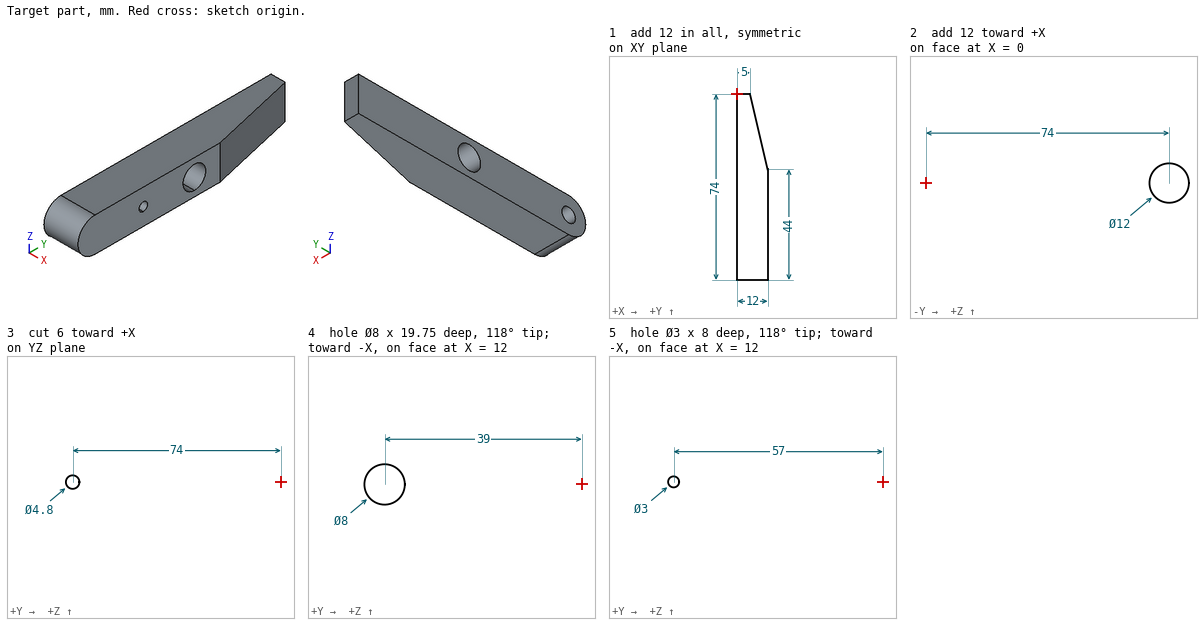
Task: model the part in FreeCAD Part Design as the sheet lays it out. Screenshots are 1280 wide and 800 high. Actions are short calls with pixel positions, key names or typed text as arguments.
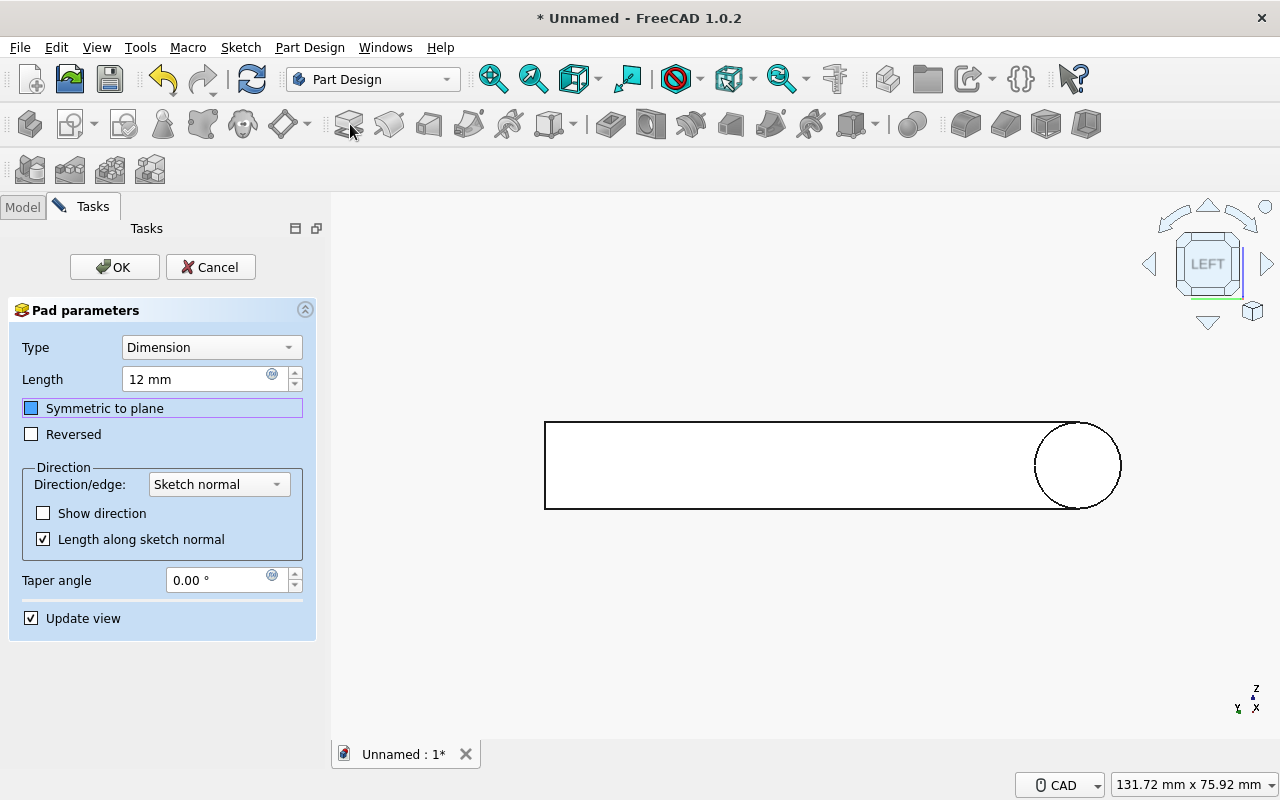
click(30, 434)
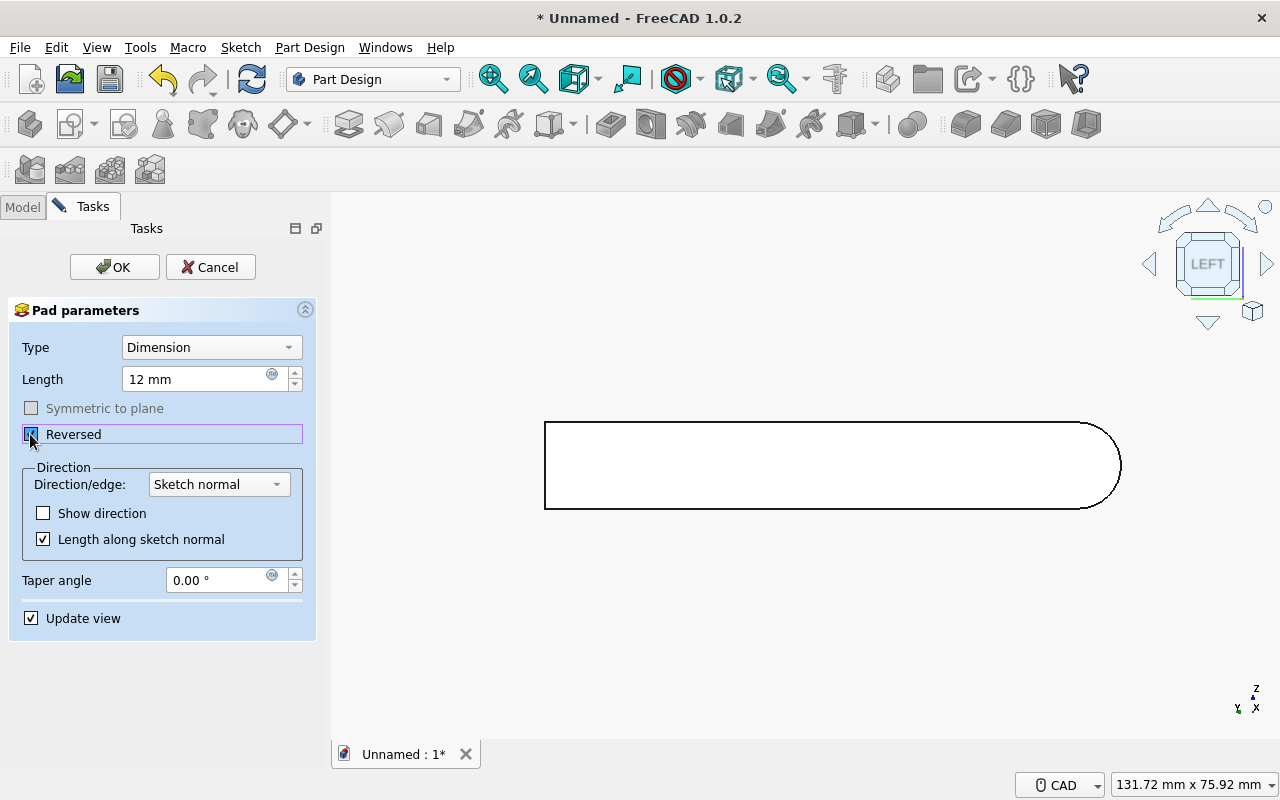
click(115, 267)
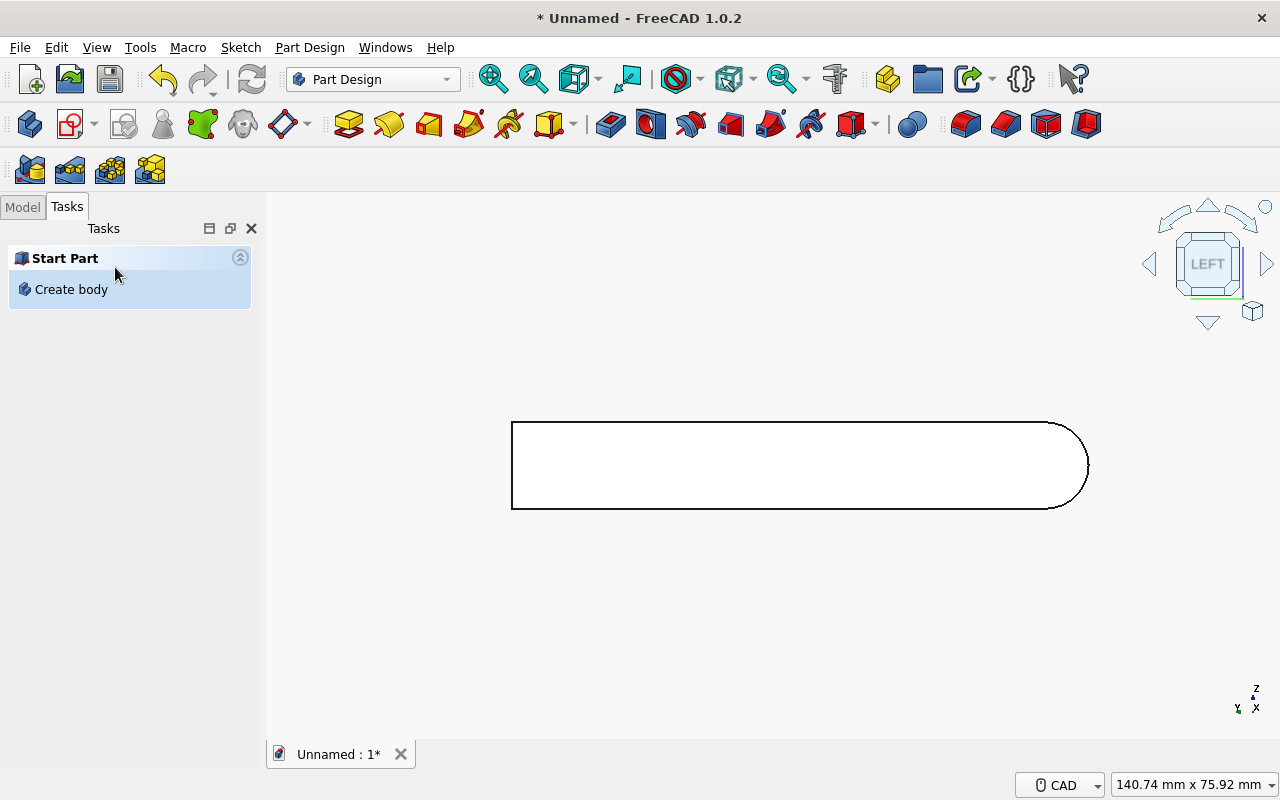
click(70, 124)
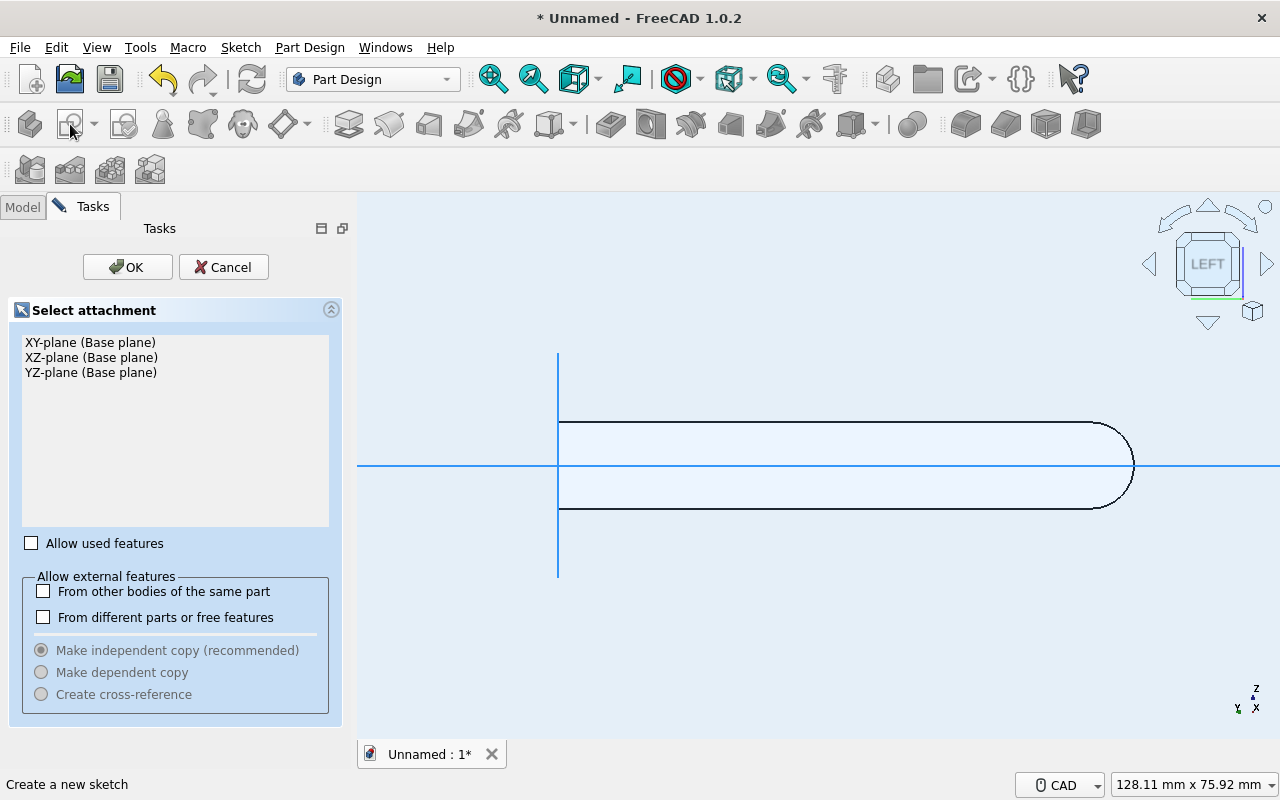
click(82, 372)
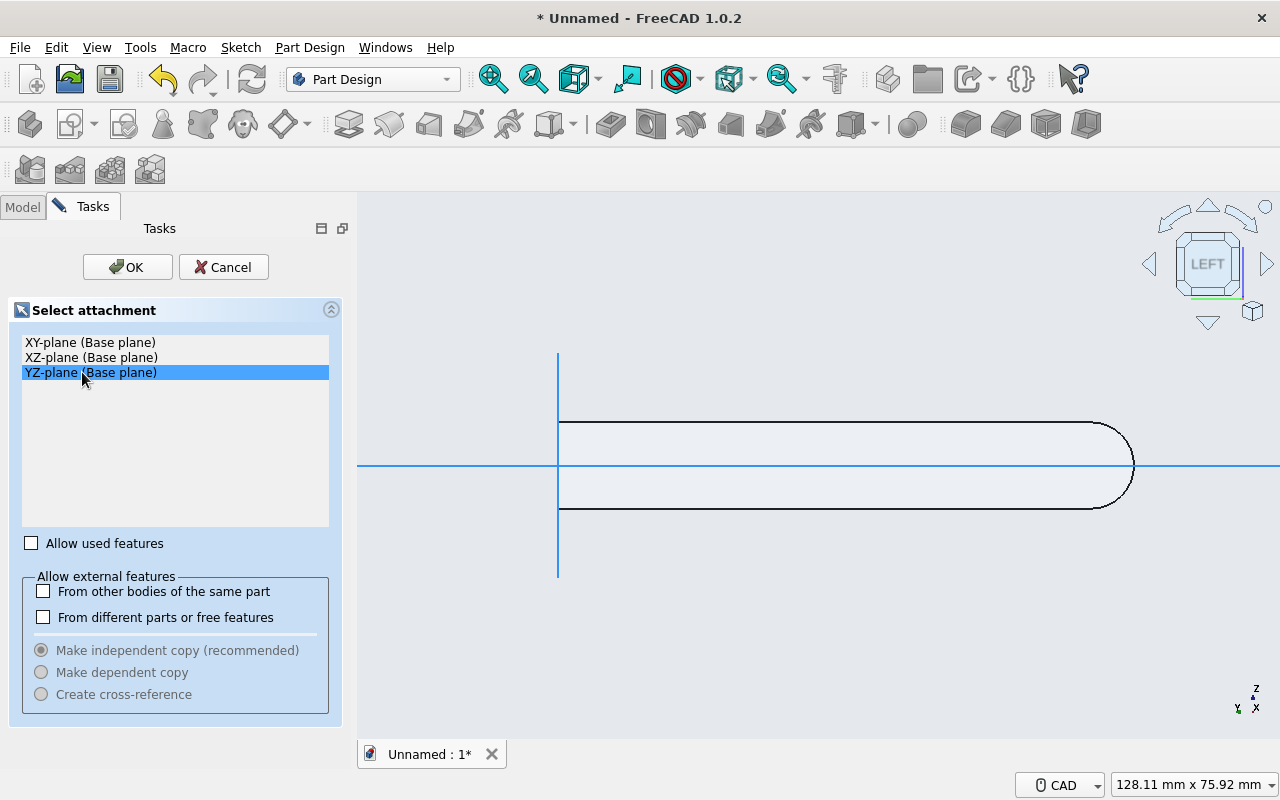
click(128, 267)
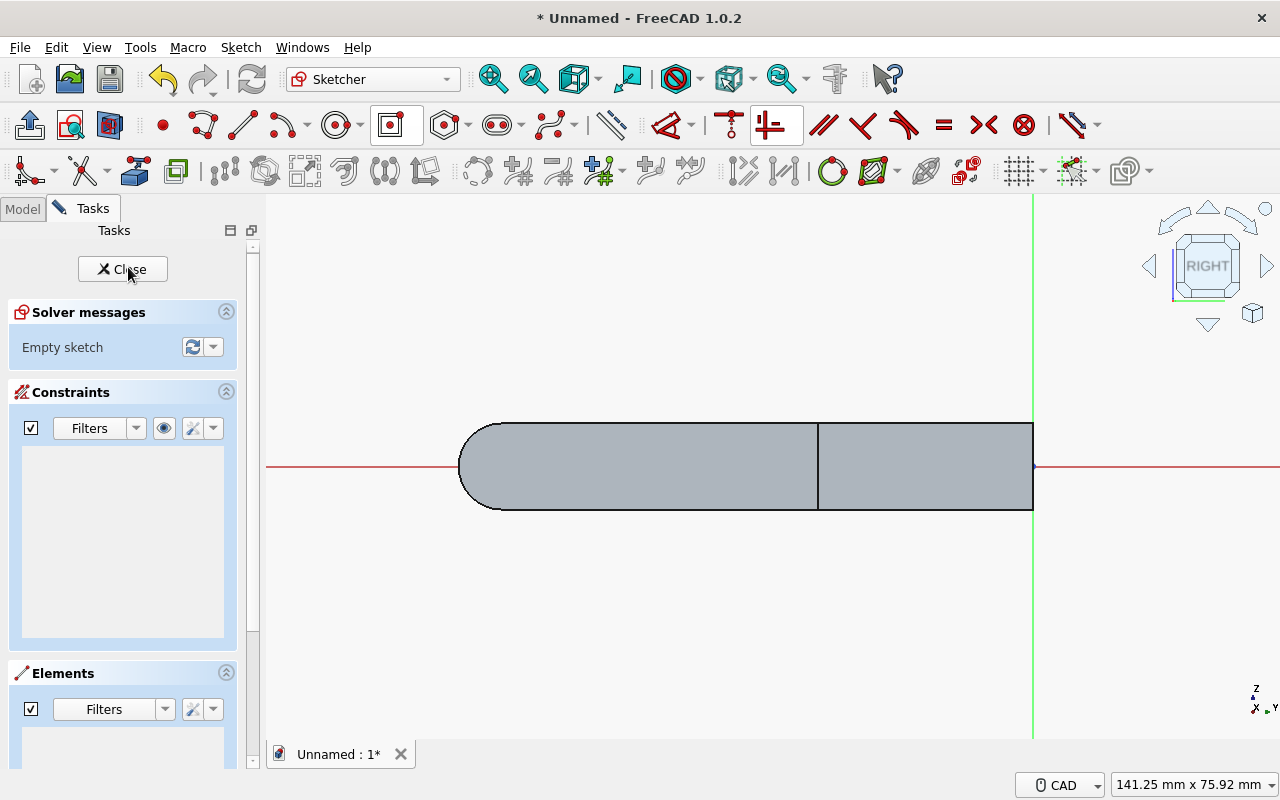
click(110, 126)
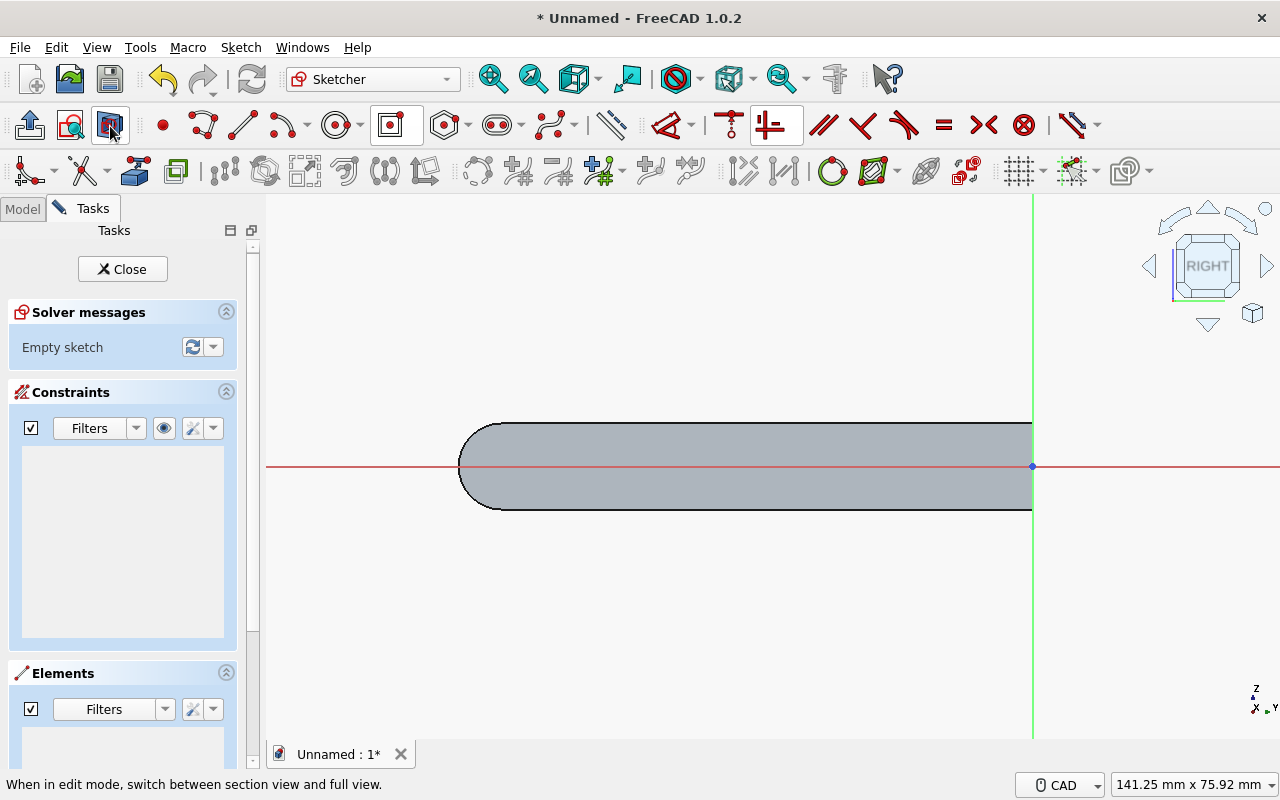
scroll(481, 467, up, 12)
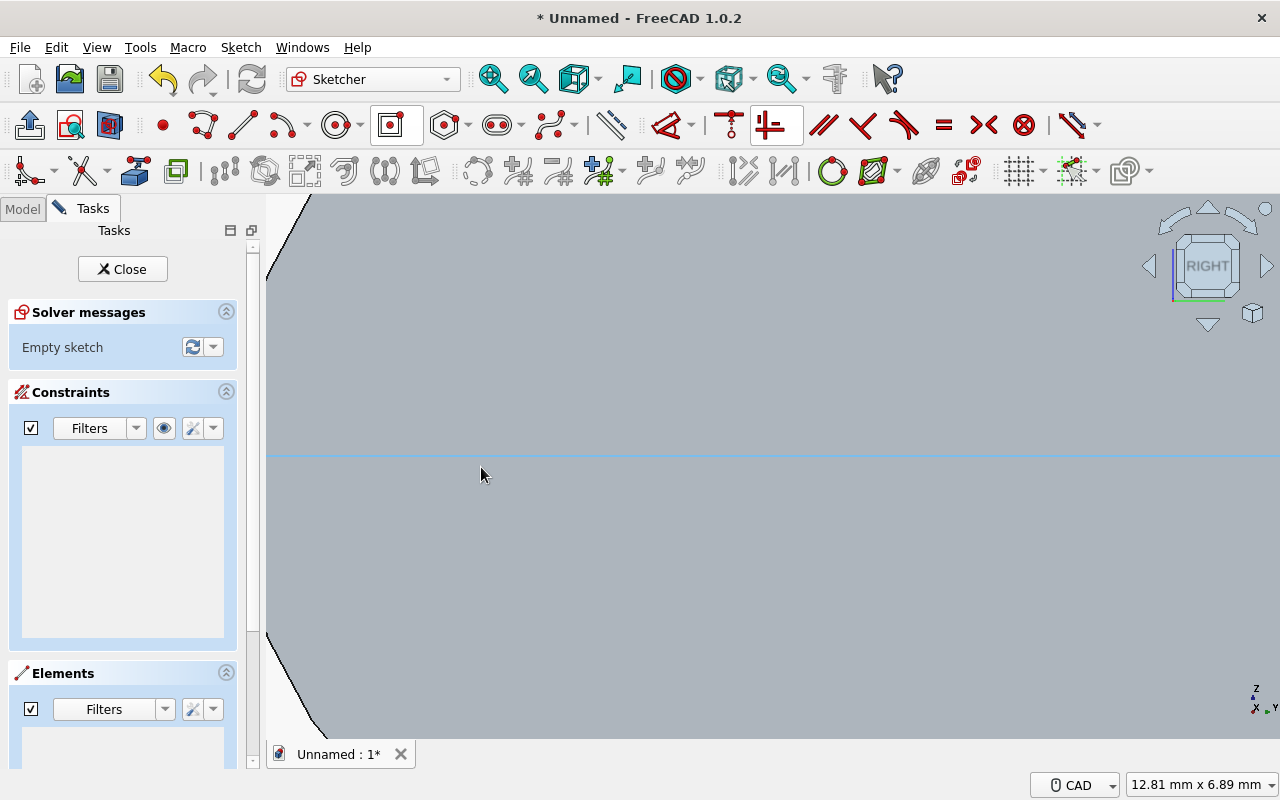
click(336, 126)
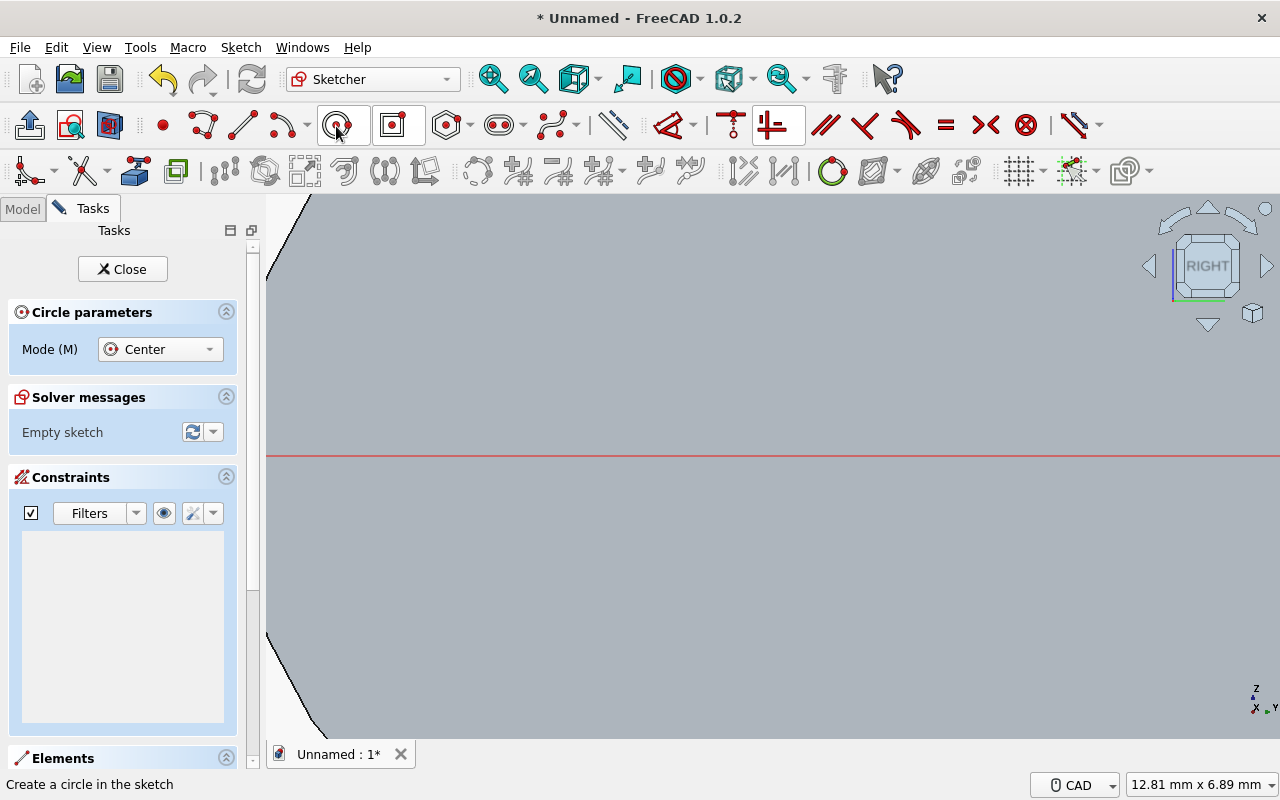
click(707, 456)
move(841, 322)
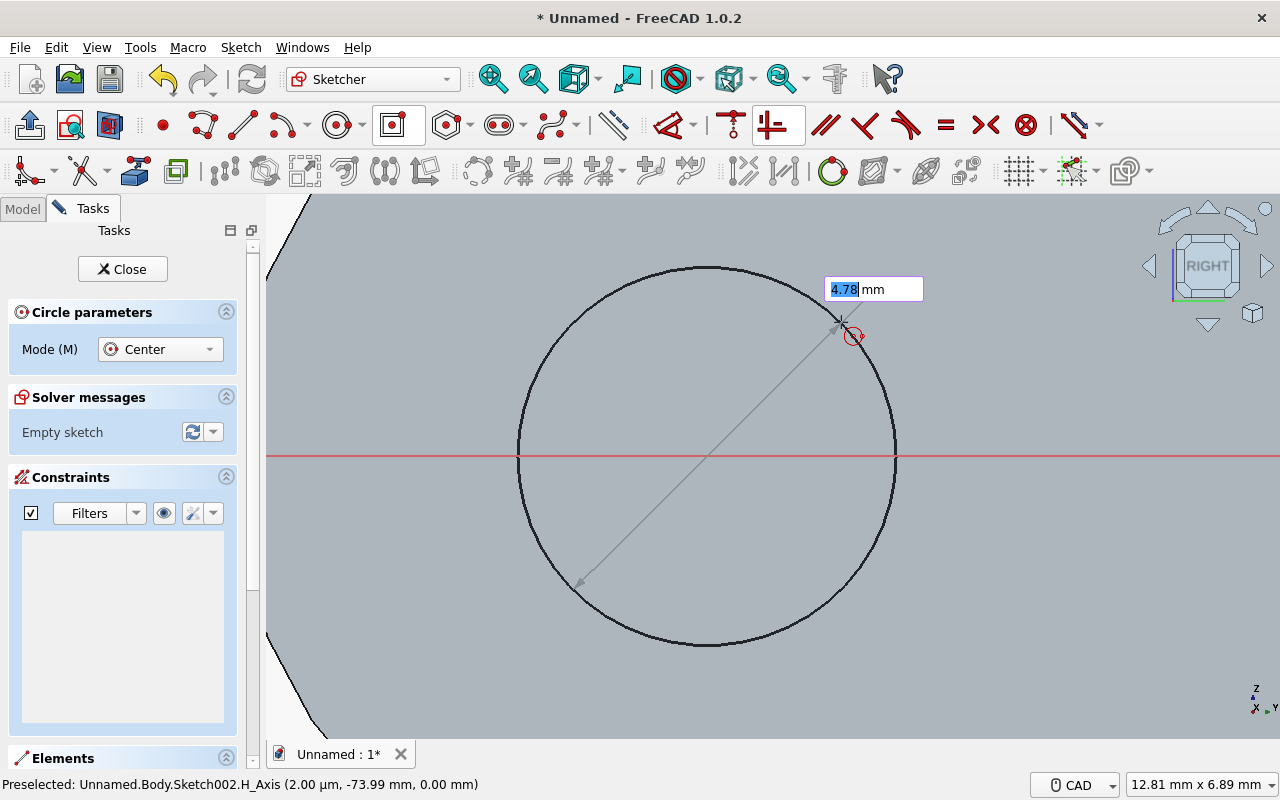
text(4.8)
key(Return)
key(Escape)